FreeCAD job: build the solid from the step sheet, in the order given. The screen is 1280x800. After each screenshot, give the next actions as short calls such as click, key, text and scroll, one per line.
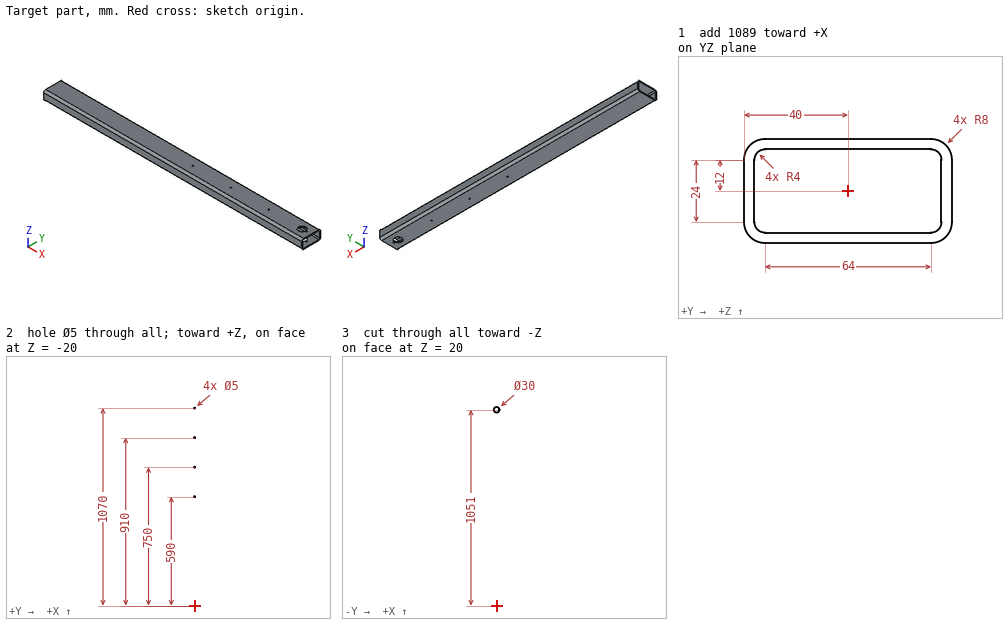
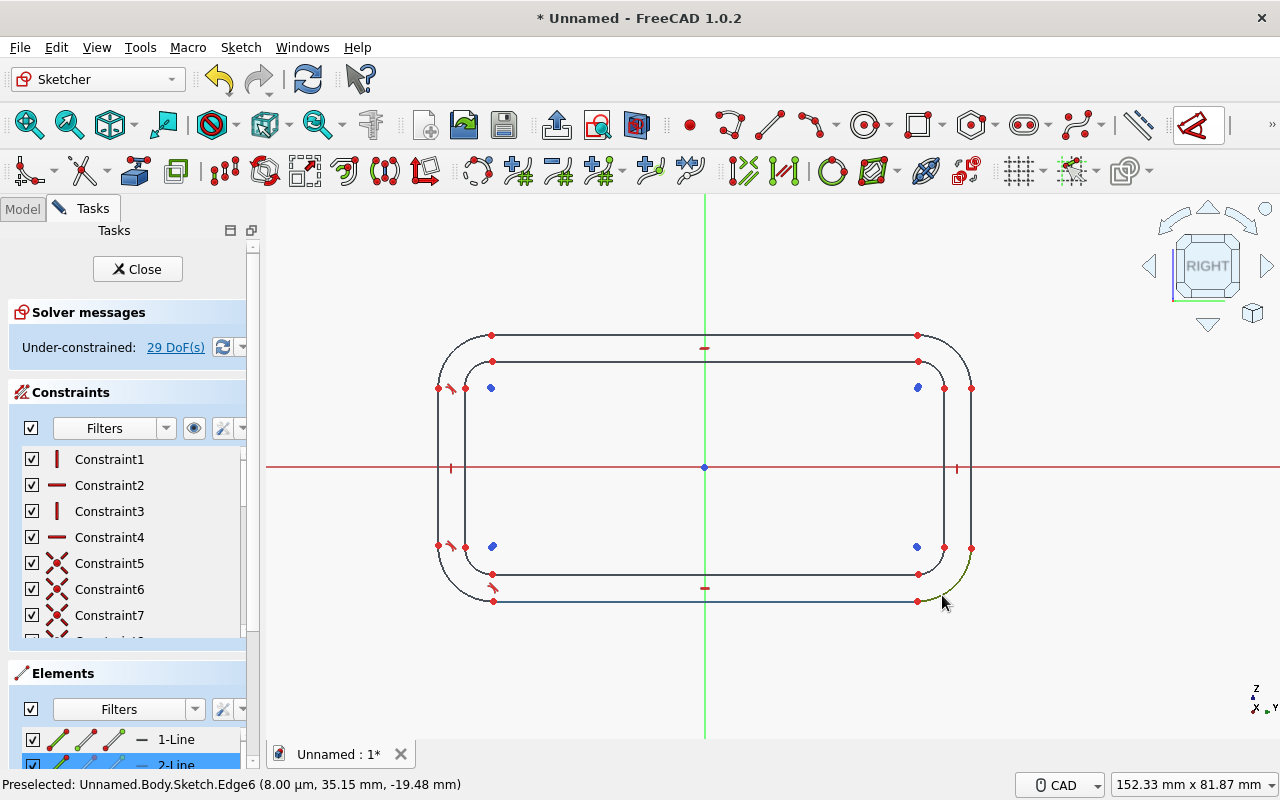
key(t)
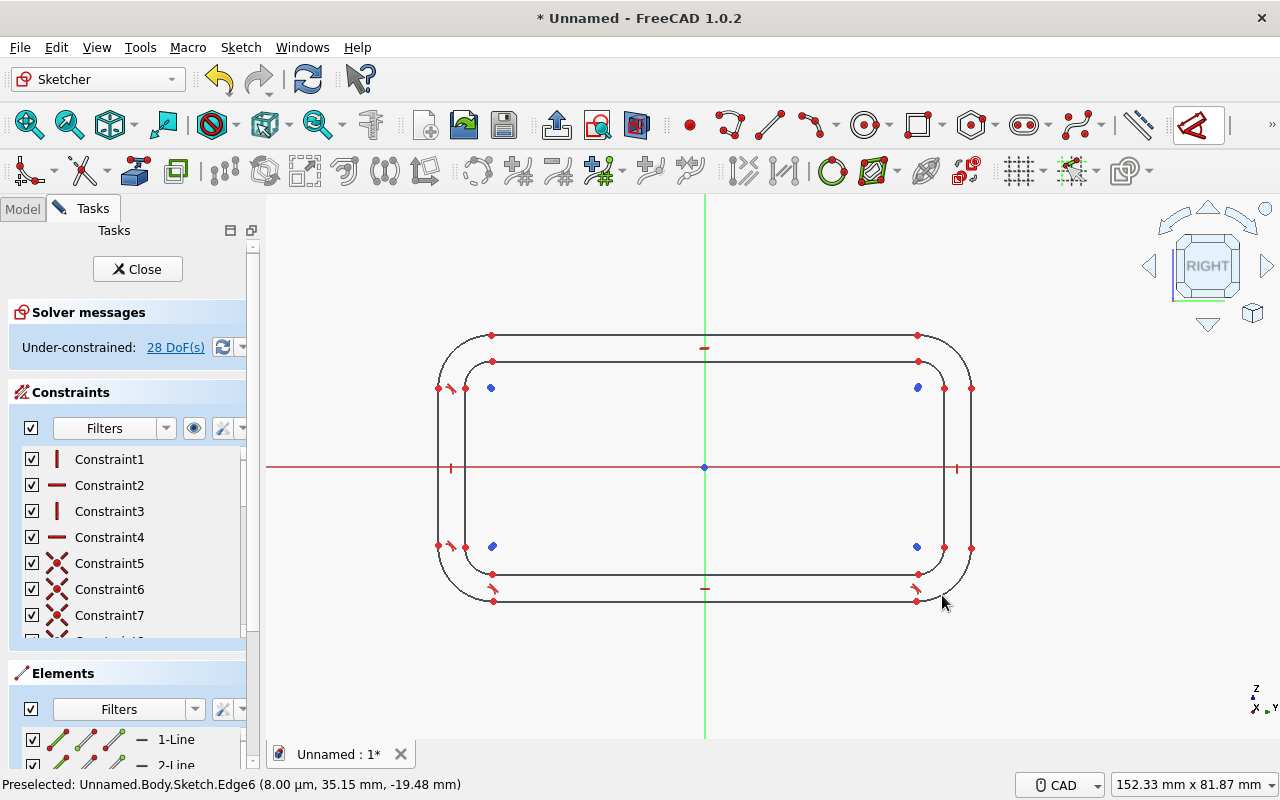
click(971, 500)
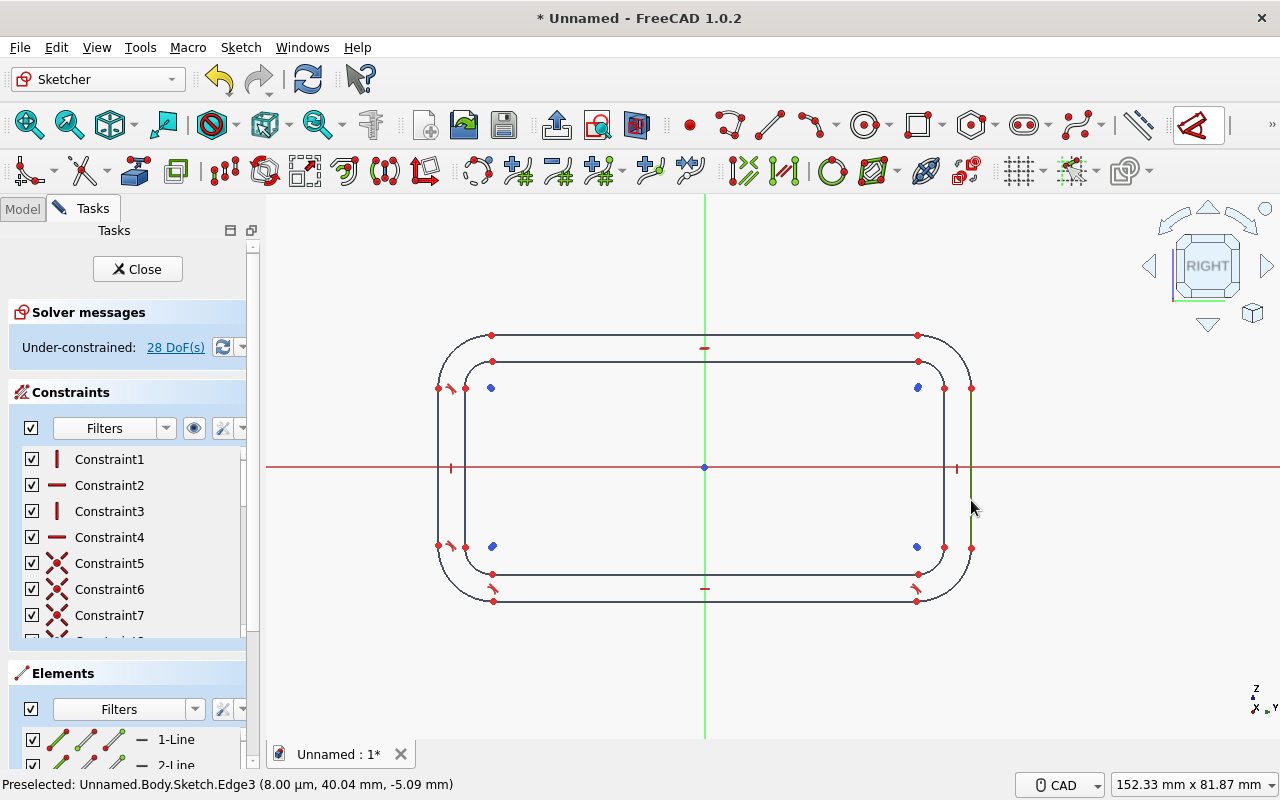
click(941, 596)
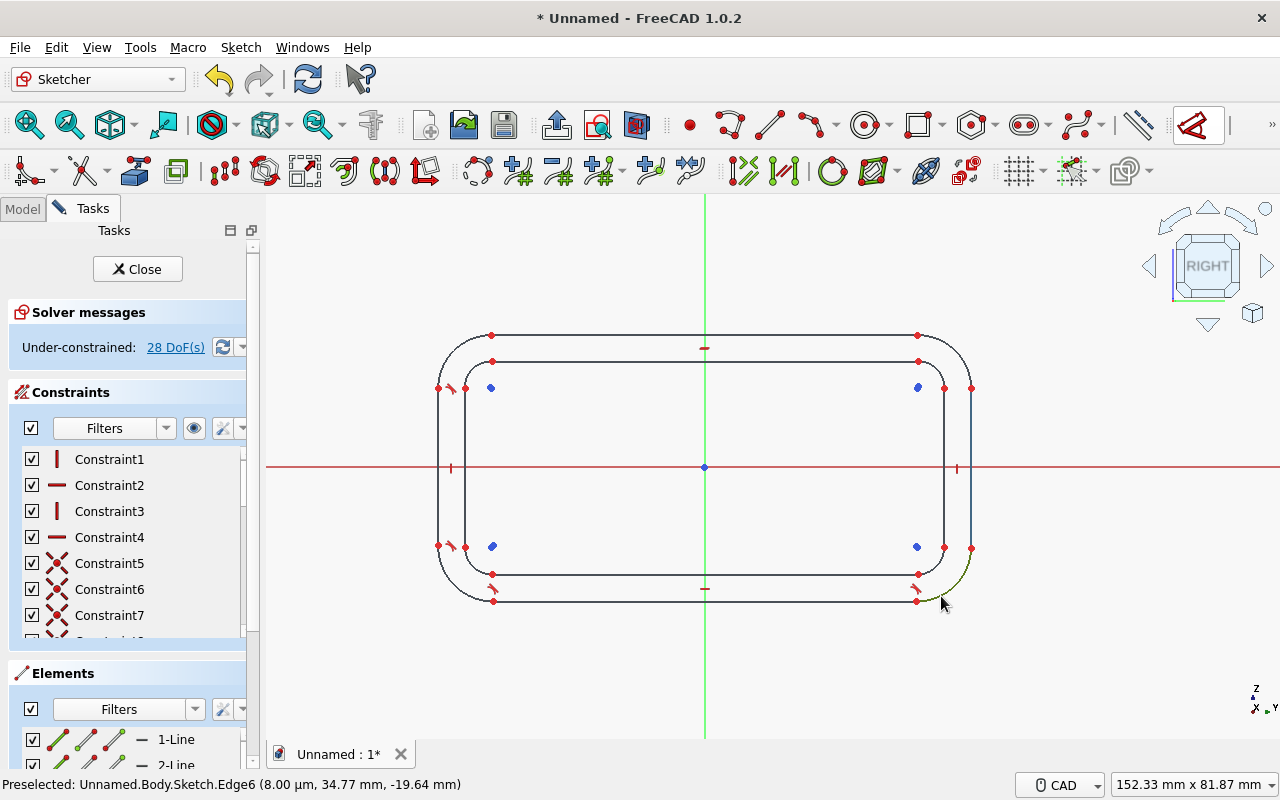
key(t)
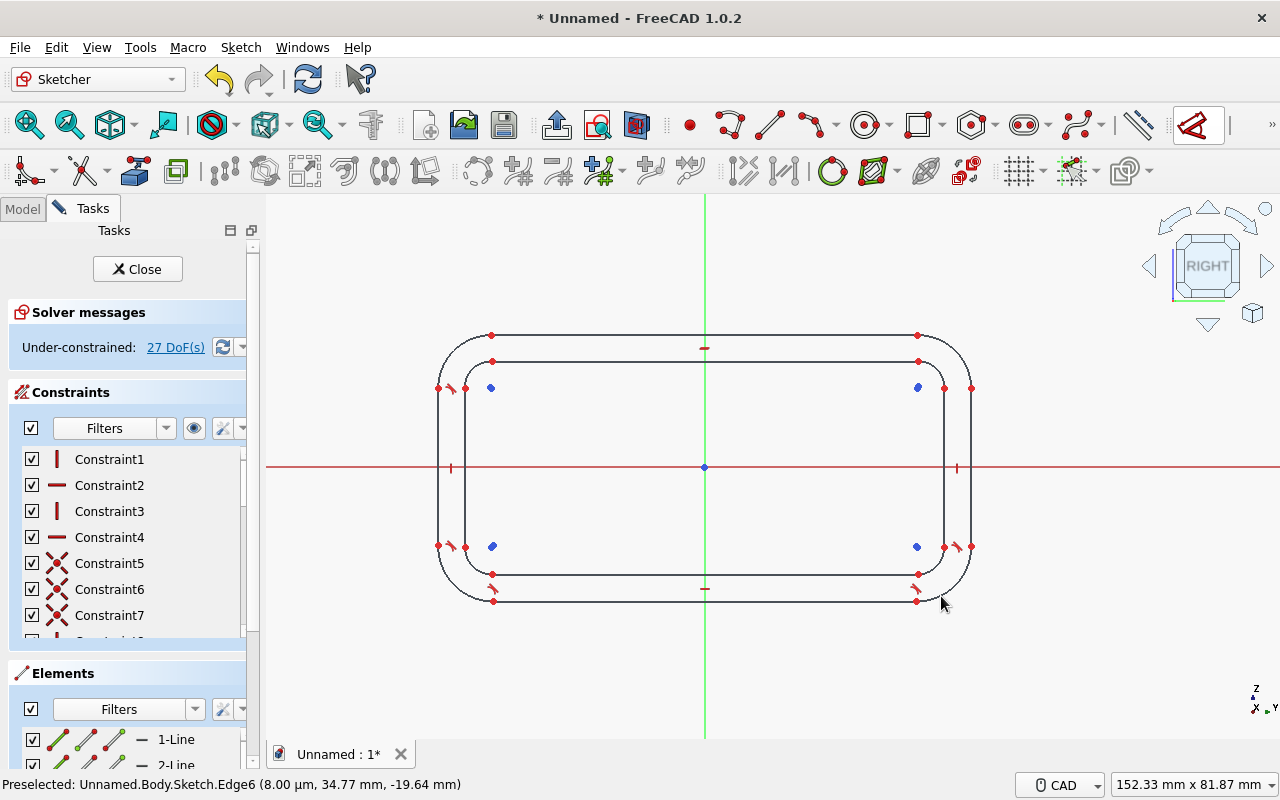
click(971, 499)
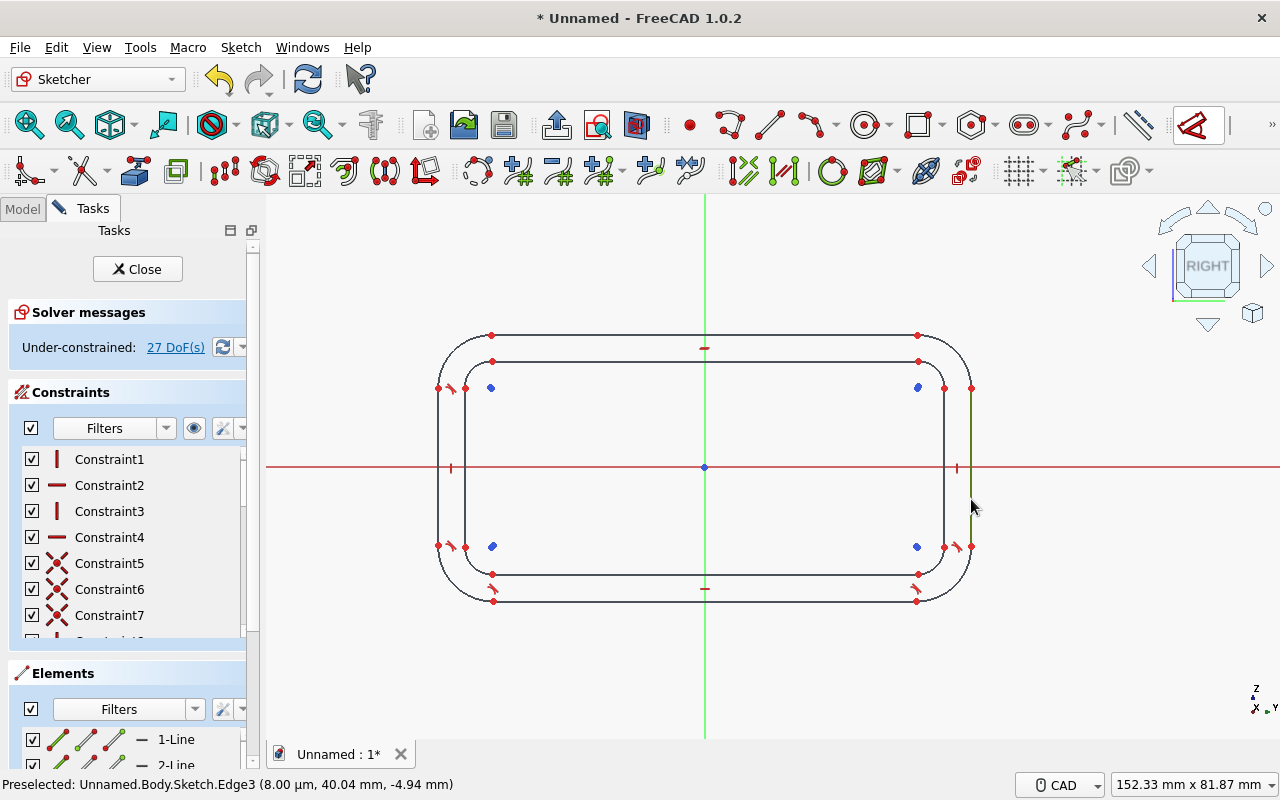
click(965, 364)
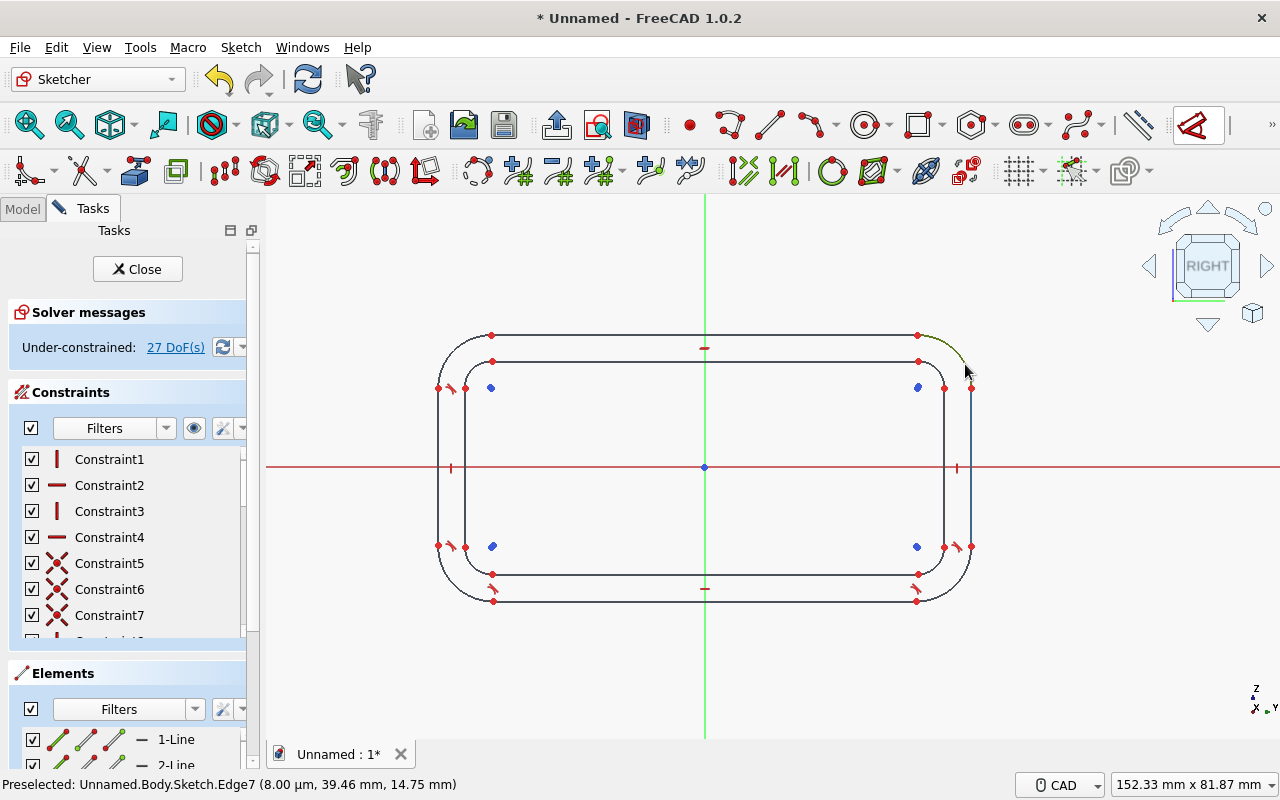
key(t)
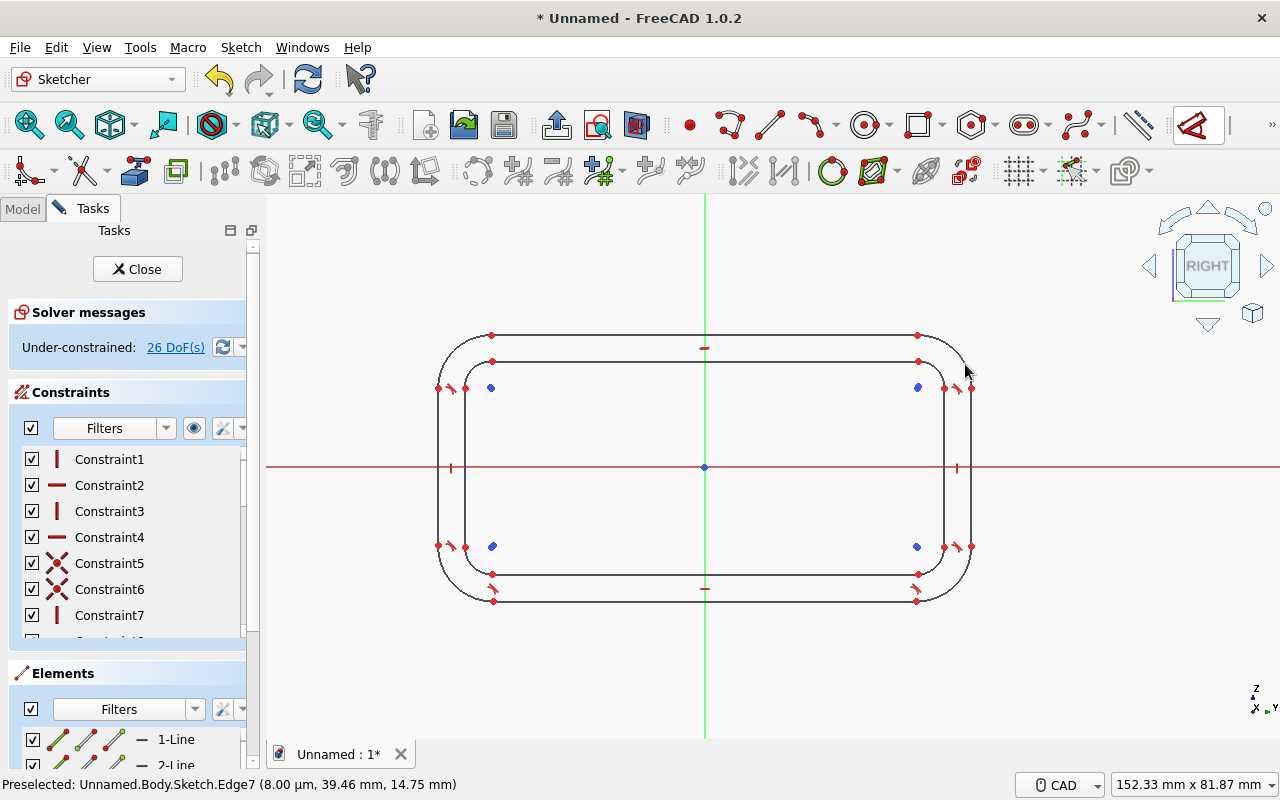
click(790, 335)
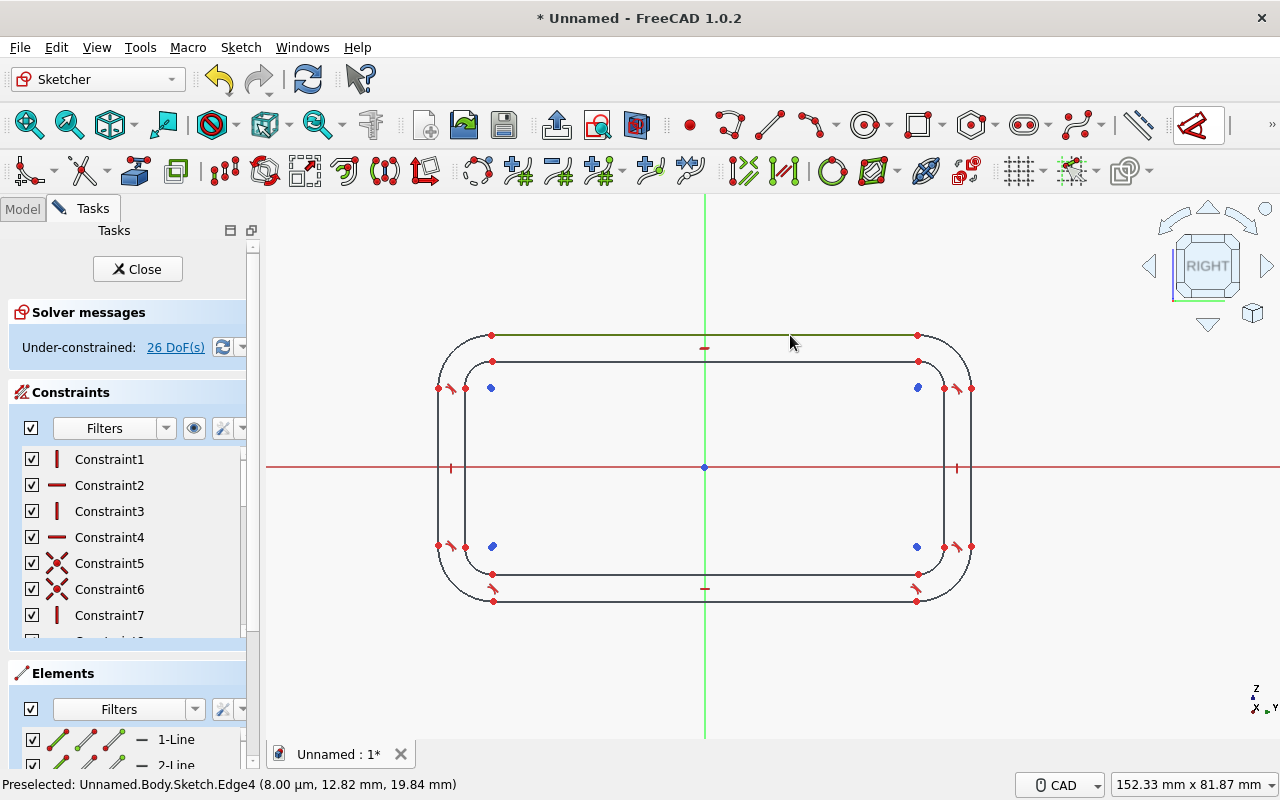
click(965, 365)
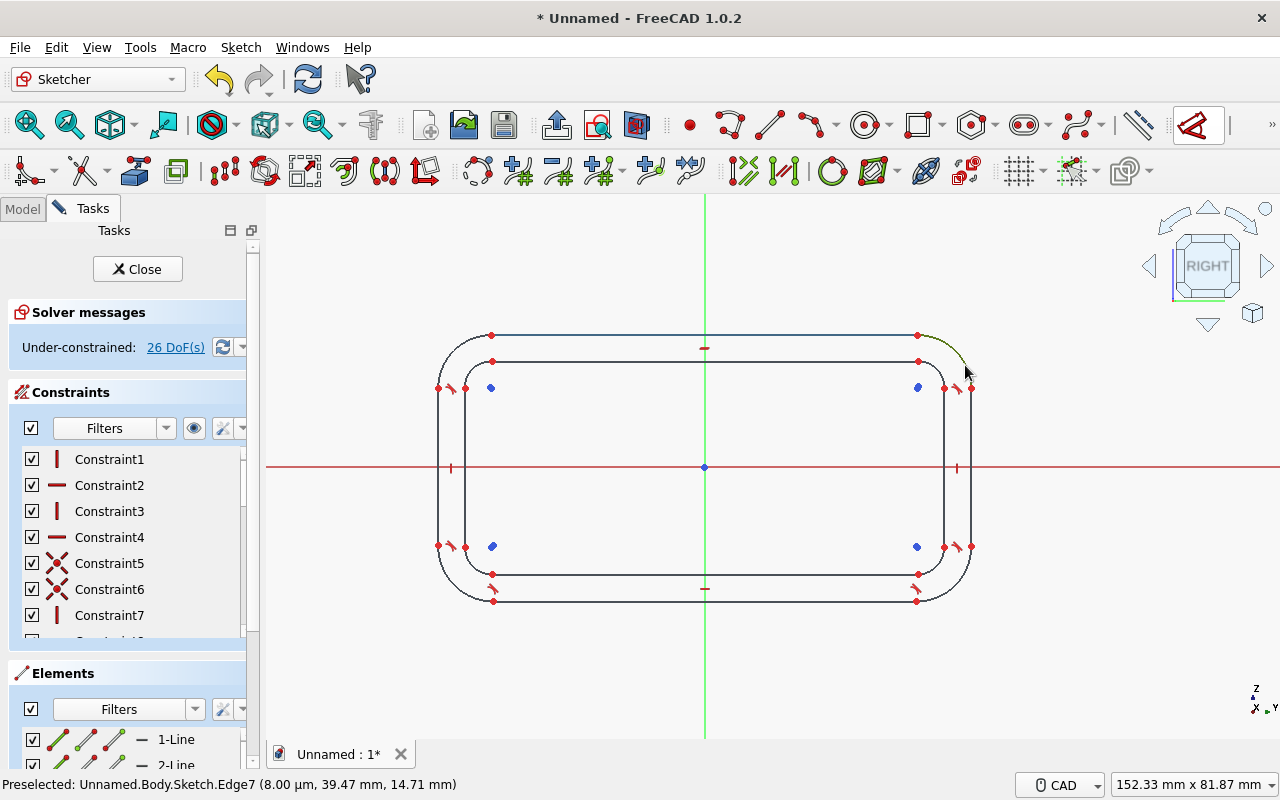
key(t)